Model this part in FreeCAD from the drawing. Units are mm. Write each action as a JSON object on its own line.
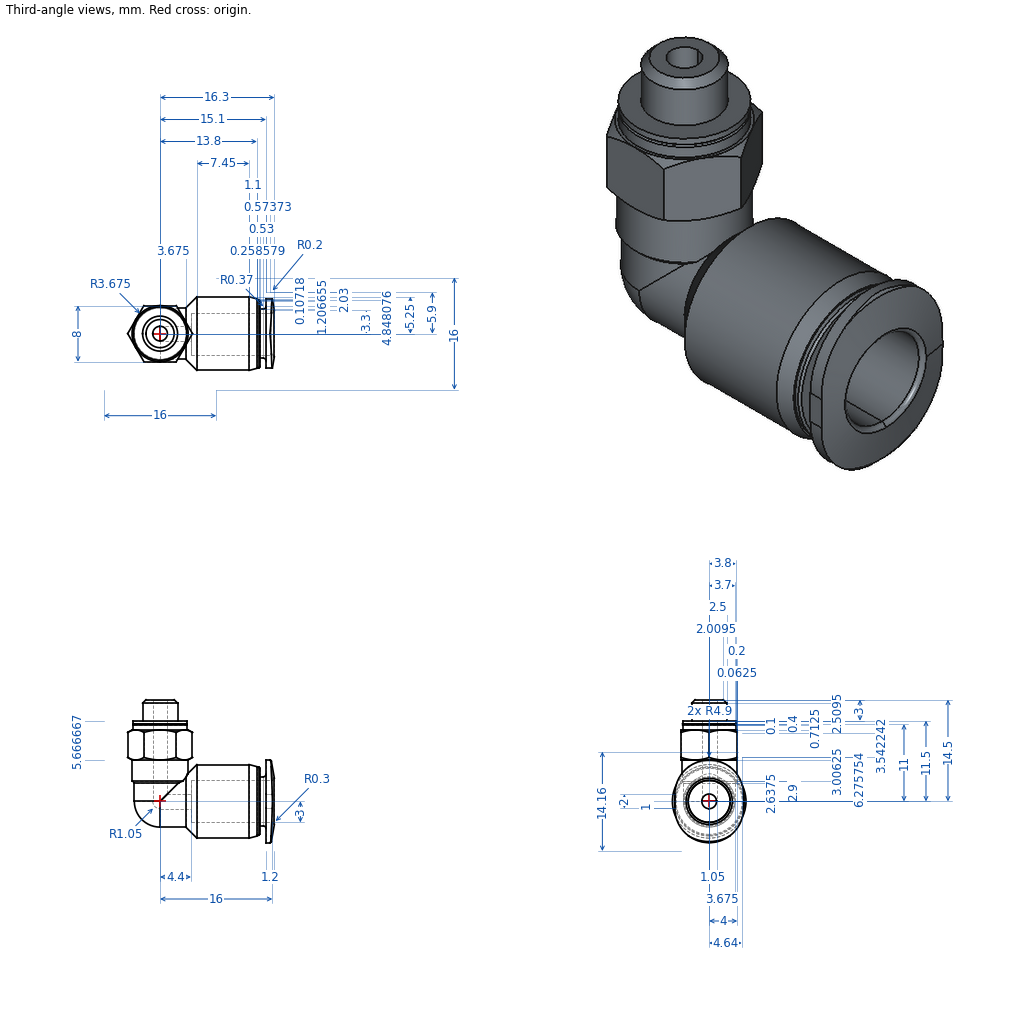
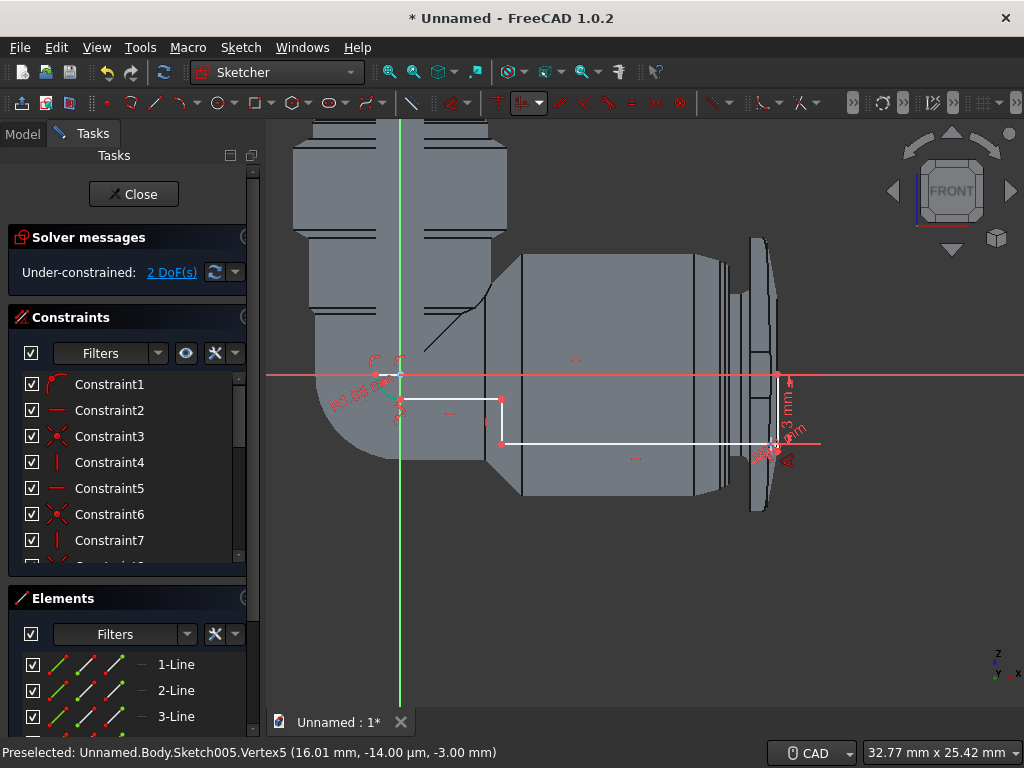
{"action": "left_click", "coordinate": [471, 399]}
{"action": "left_click", "coordinate": [451, 433]}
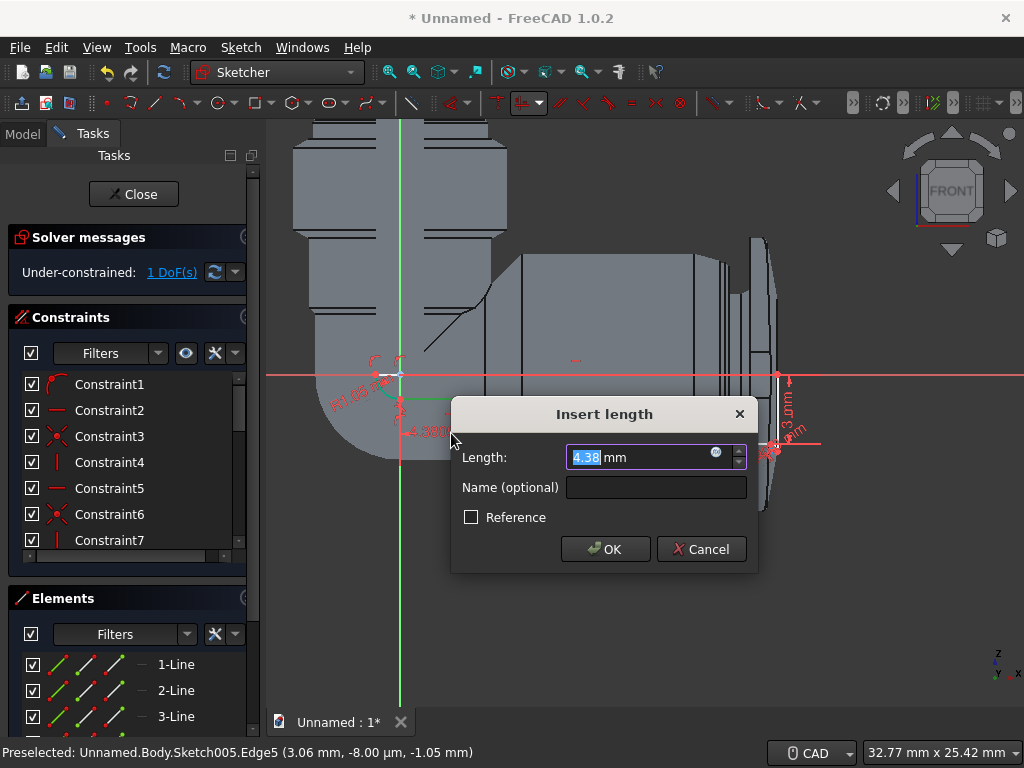
{"action": "type", "text": "4.4"}
{"action": "key", "text": "Return"}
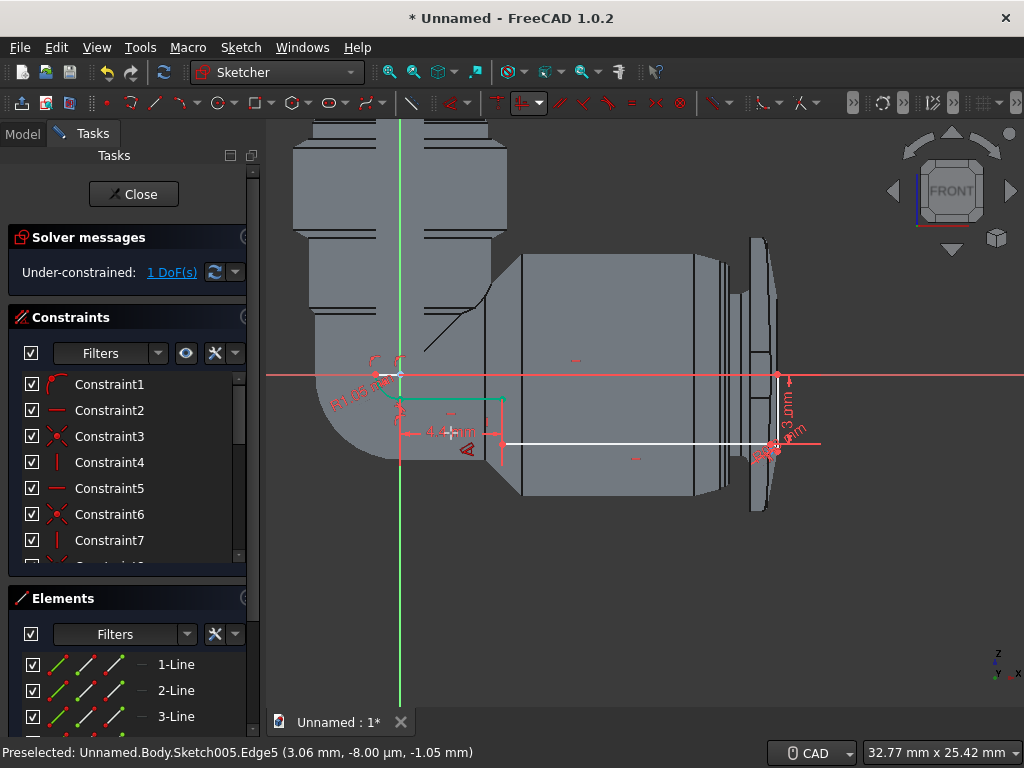
{"action": "scroll", "coordinate": [771, 444], "scroll_direction": "up", "scroll_amount": 3}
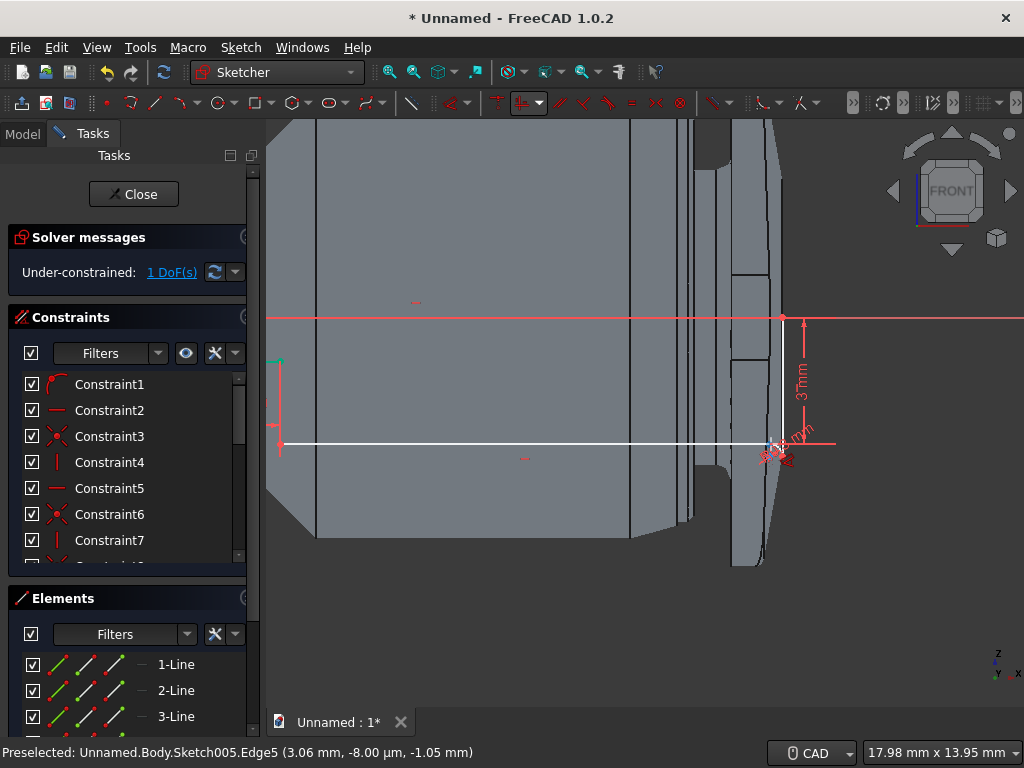
{"action": "left_click", "coordinate": [770, 444]}
{"action": "left_click", "coordinate": [532, 284]}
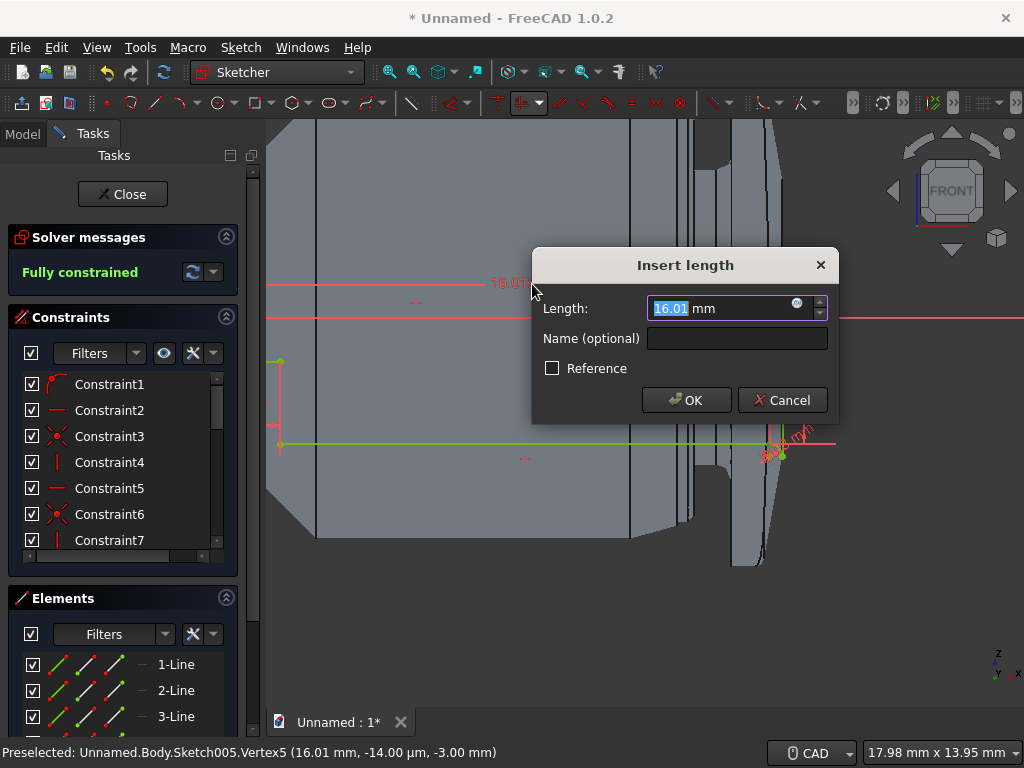
{"action": "type", "text": "16"}
{"action": "key", "text": "Return"}
{"action": "key", "text": "Escape"}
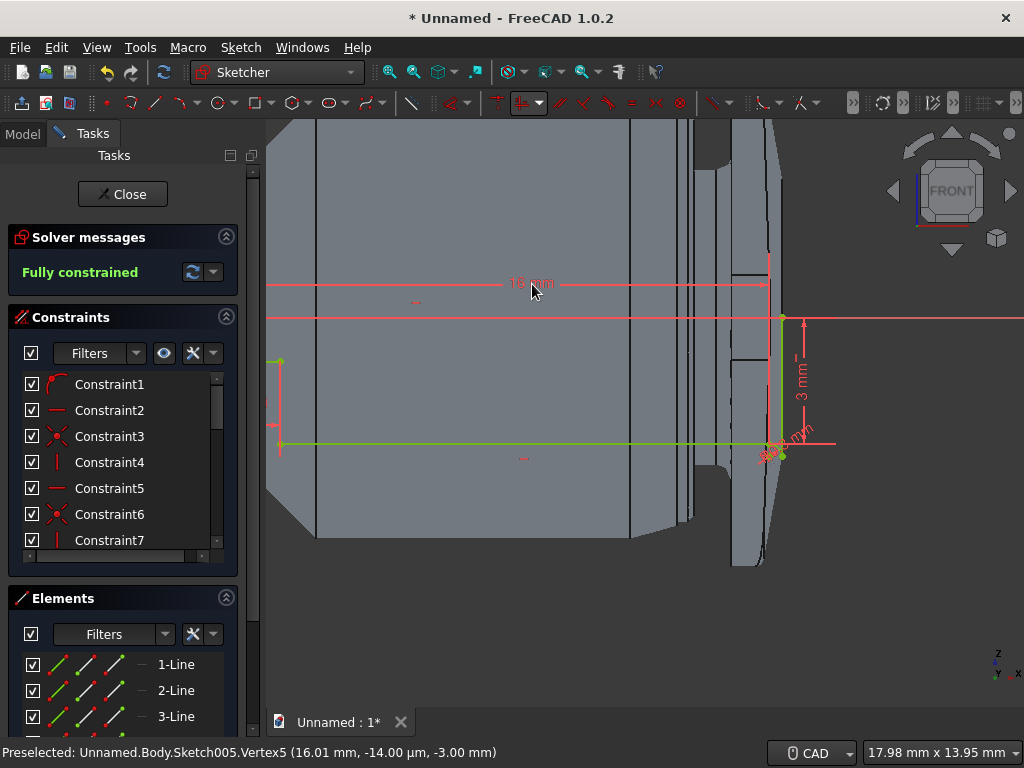
{"action": "left_click", "coordinate": [123, 194]}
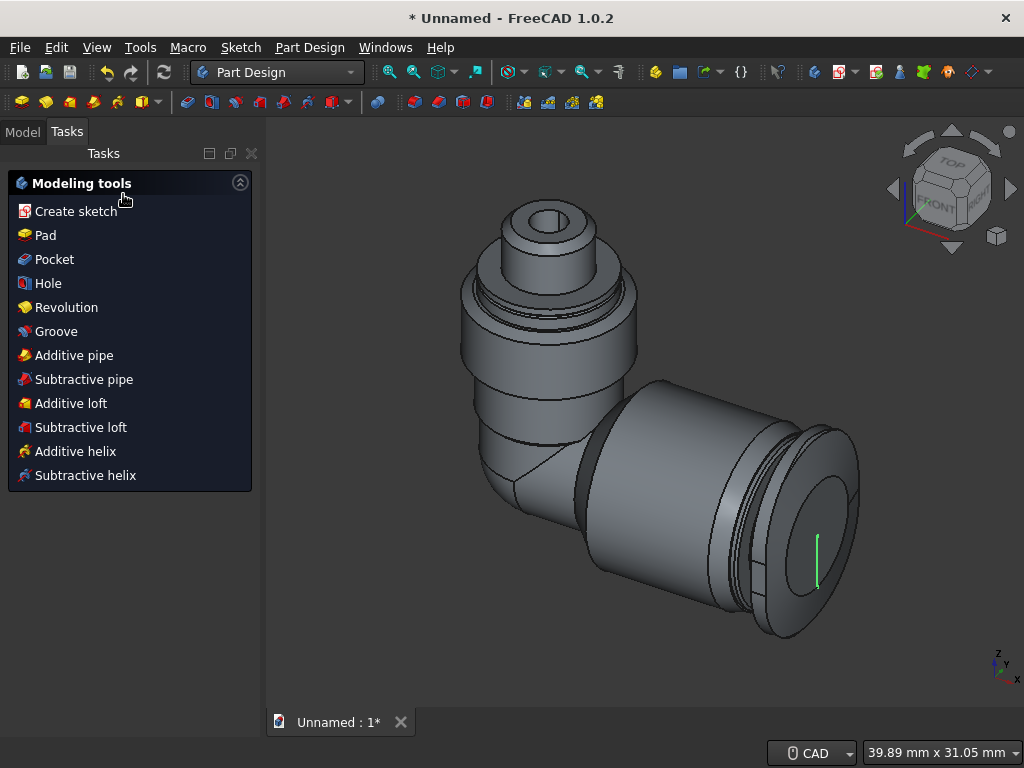
{"action": "left_click", "coordinate": [236, 102]}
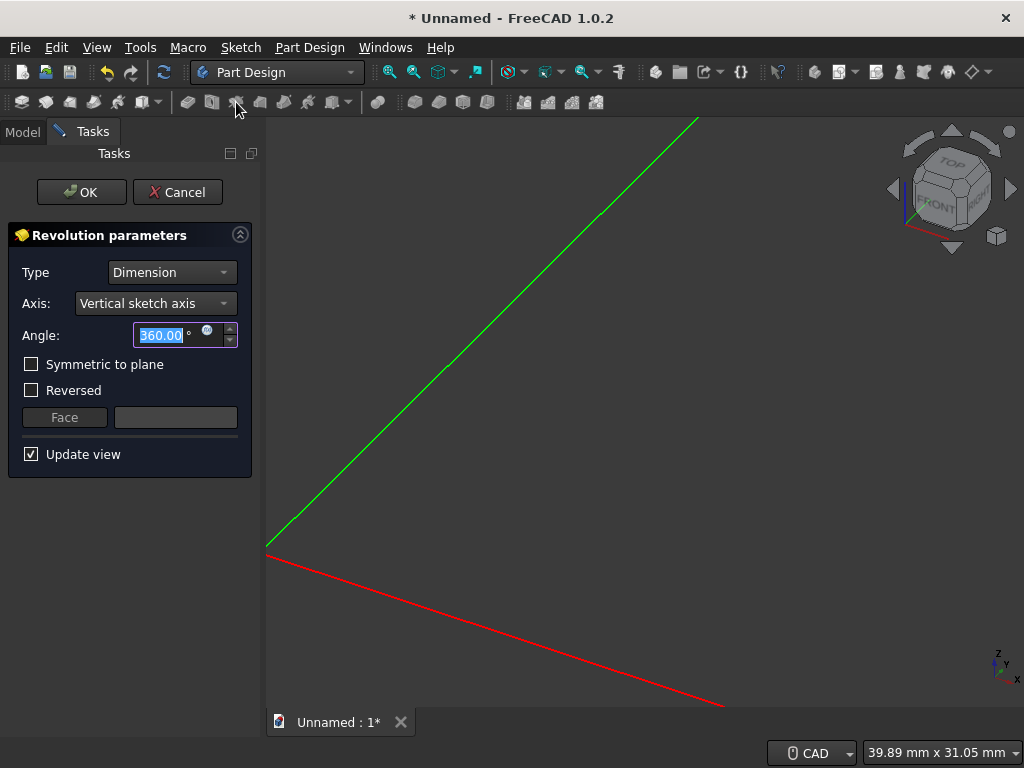
{"action": "left_click", "coordinate": [156, 304]}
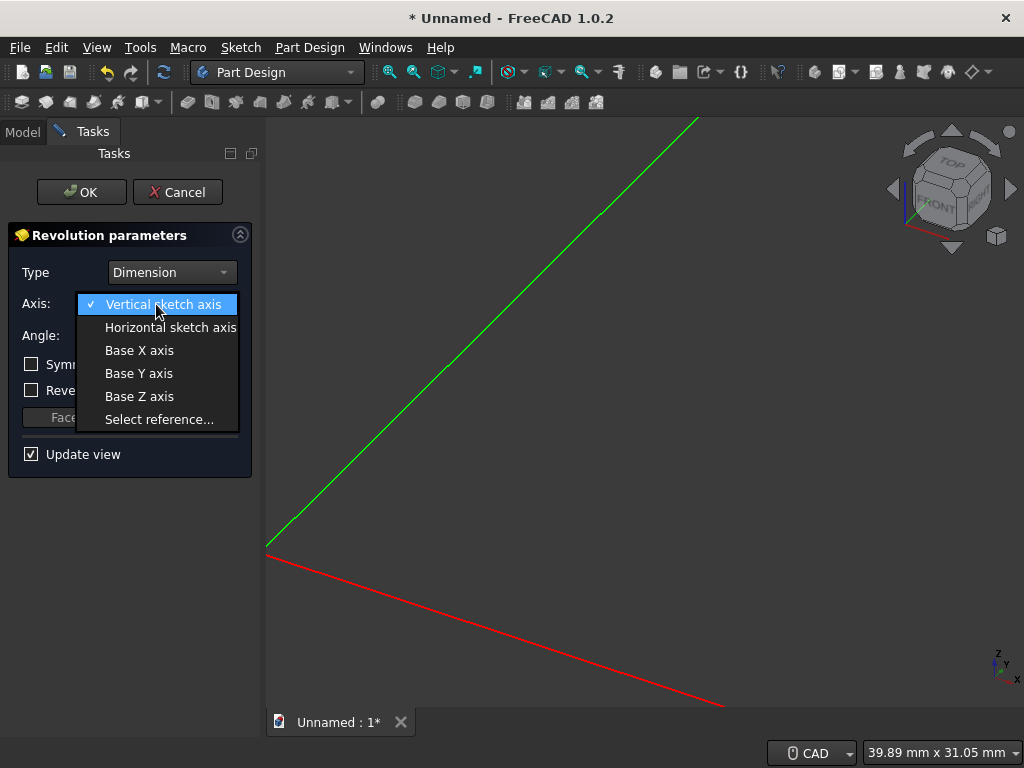
{"action": "left_click", "coordinate": [156, 328]}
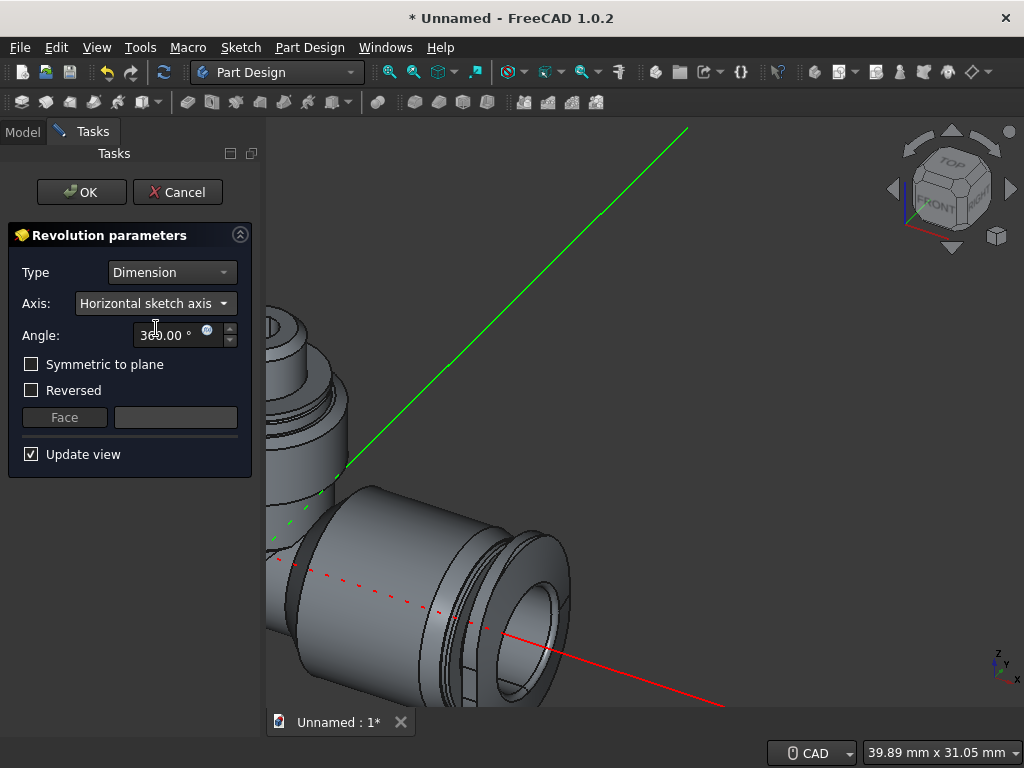
{"action": "left_click", "coordinate": [82, 192]}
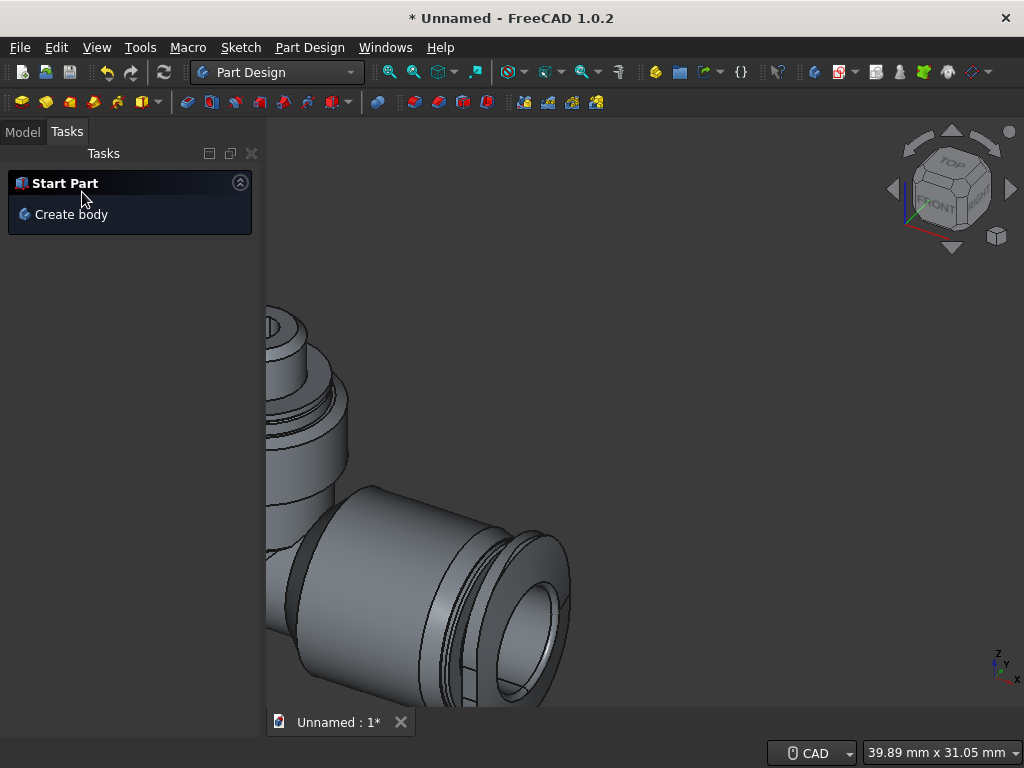
{"action": "left_click", "coordinate": [390, 72]}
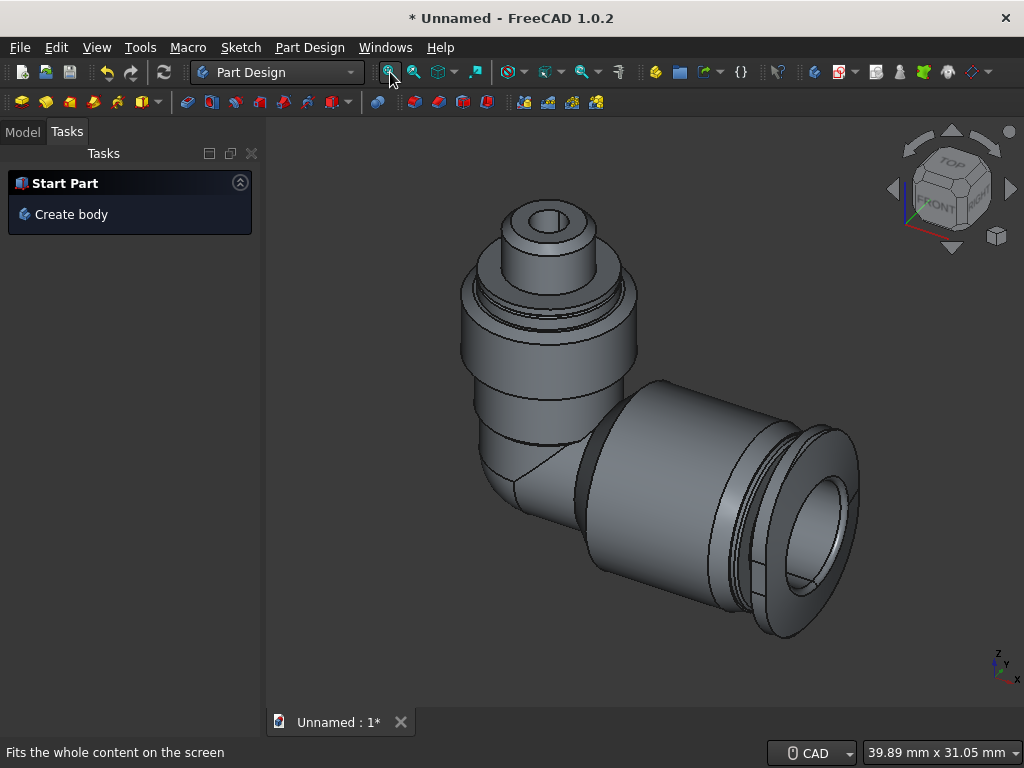
{"action": "left_click", "coordinate": [492, 276]}